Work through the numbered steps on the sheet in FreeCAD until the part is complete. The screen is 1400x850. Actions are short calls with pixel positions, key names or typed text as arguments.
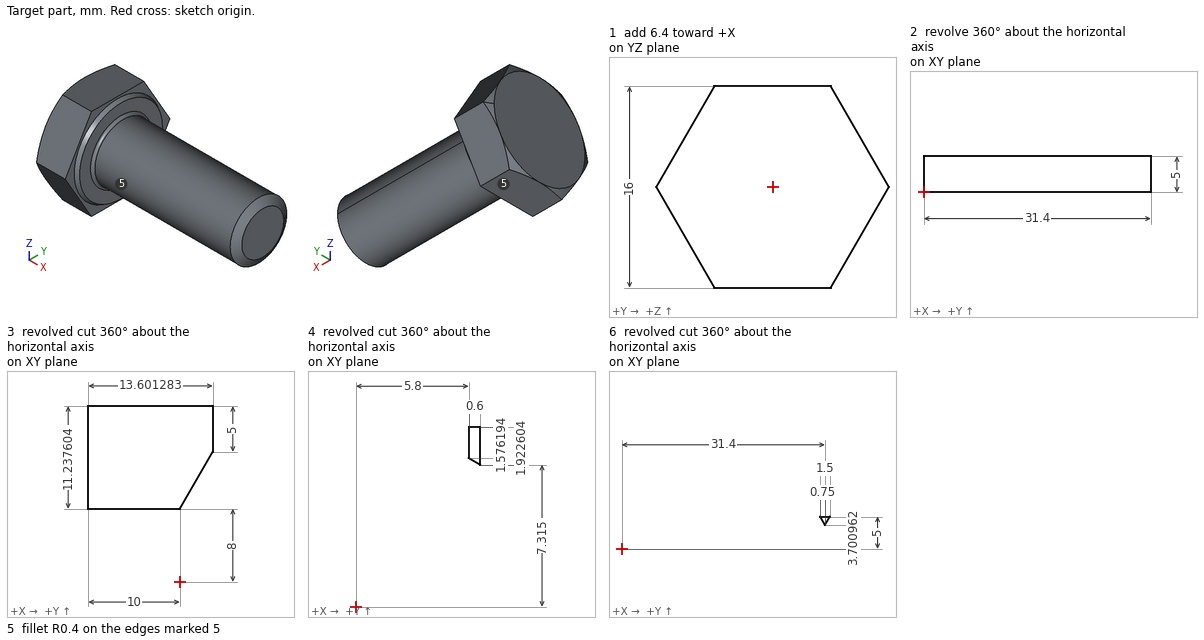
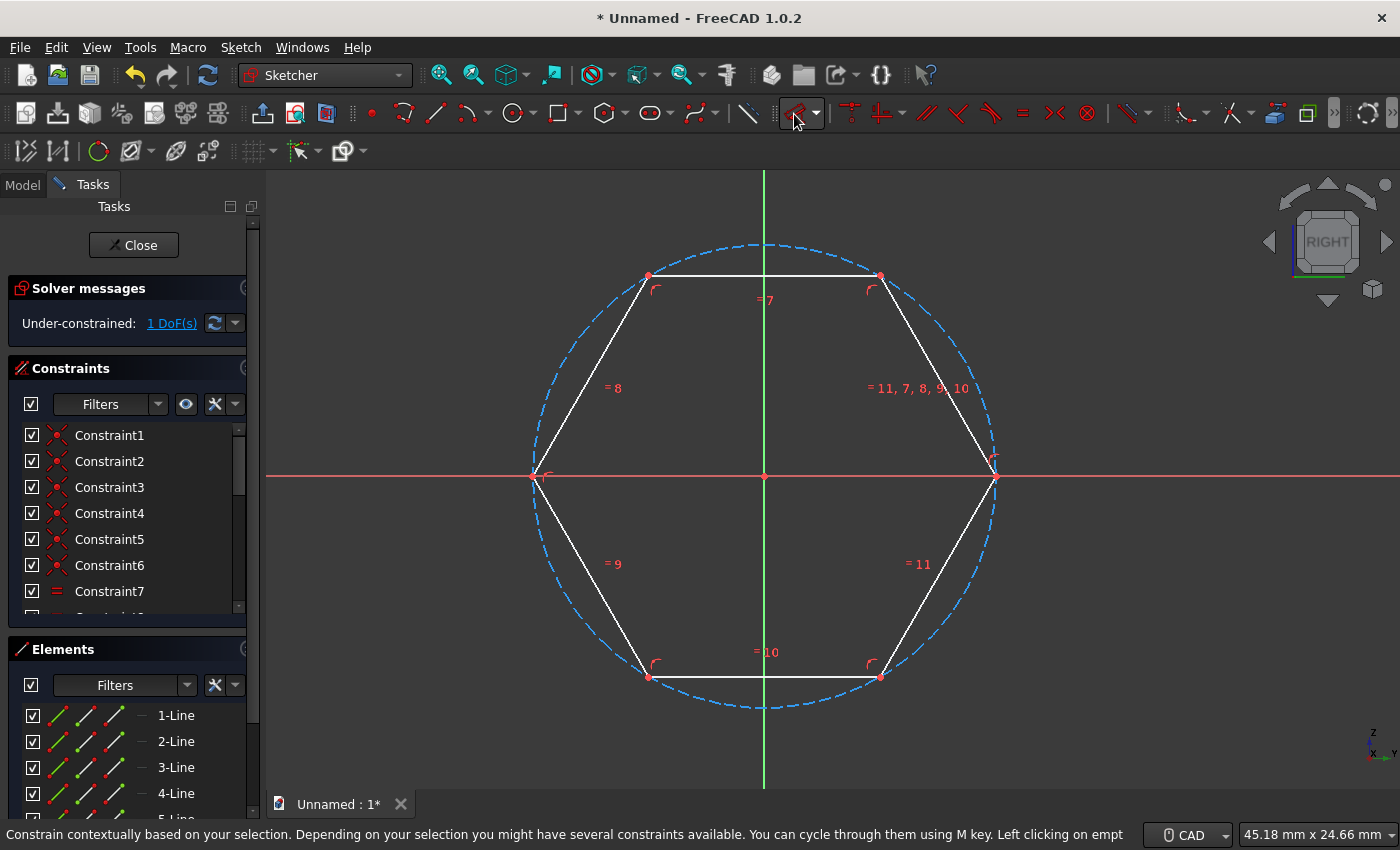
click(649, 677)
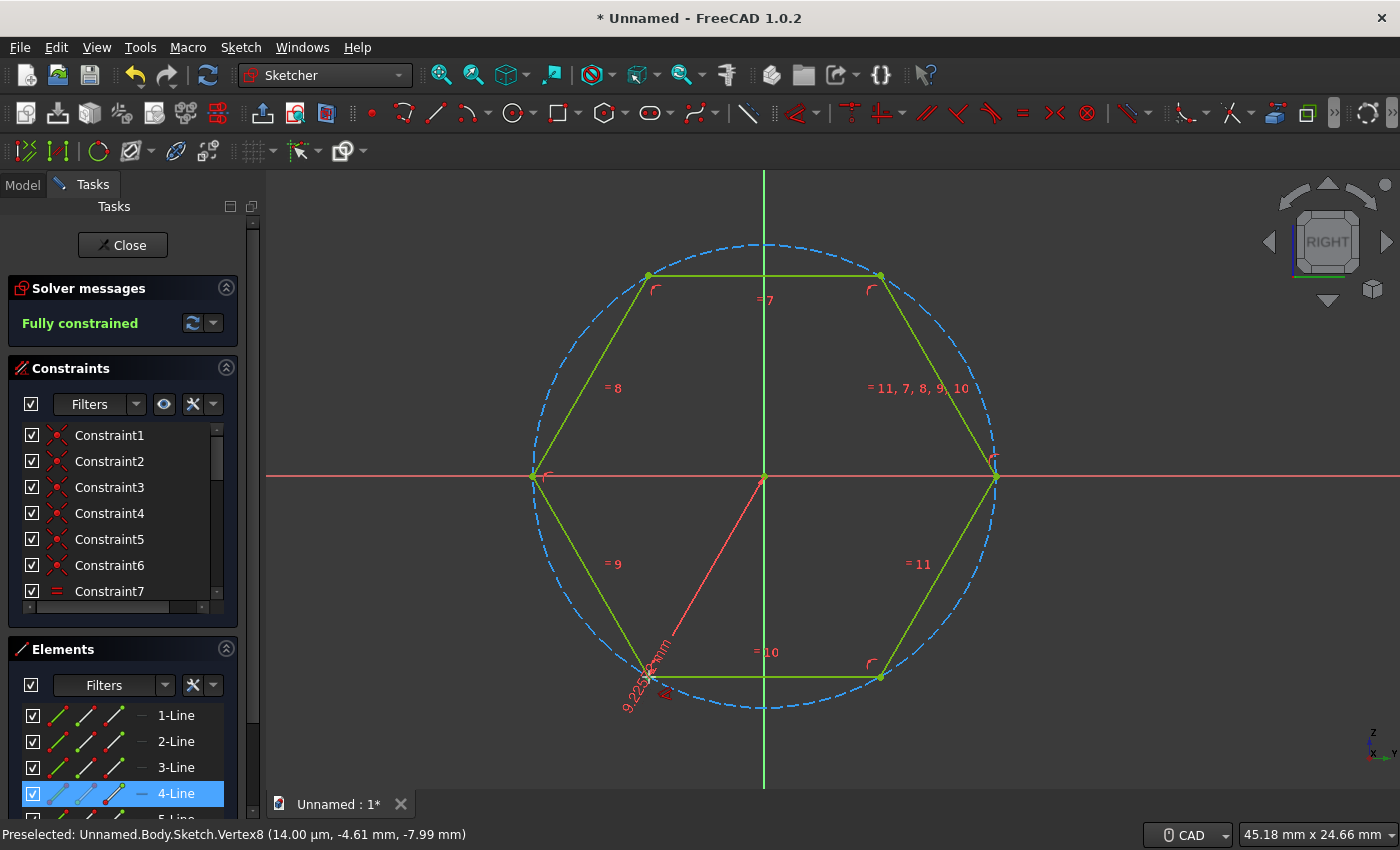
click(880, 276)
click(914, 384)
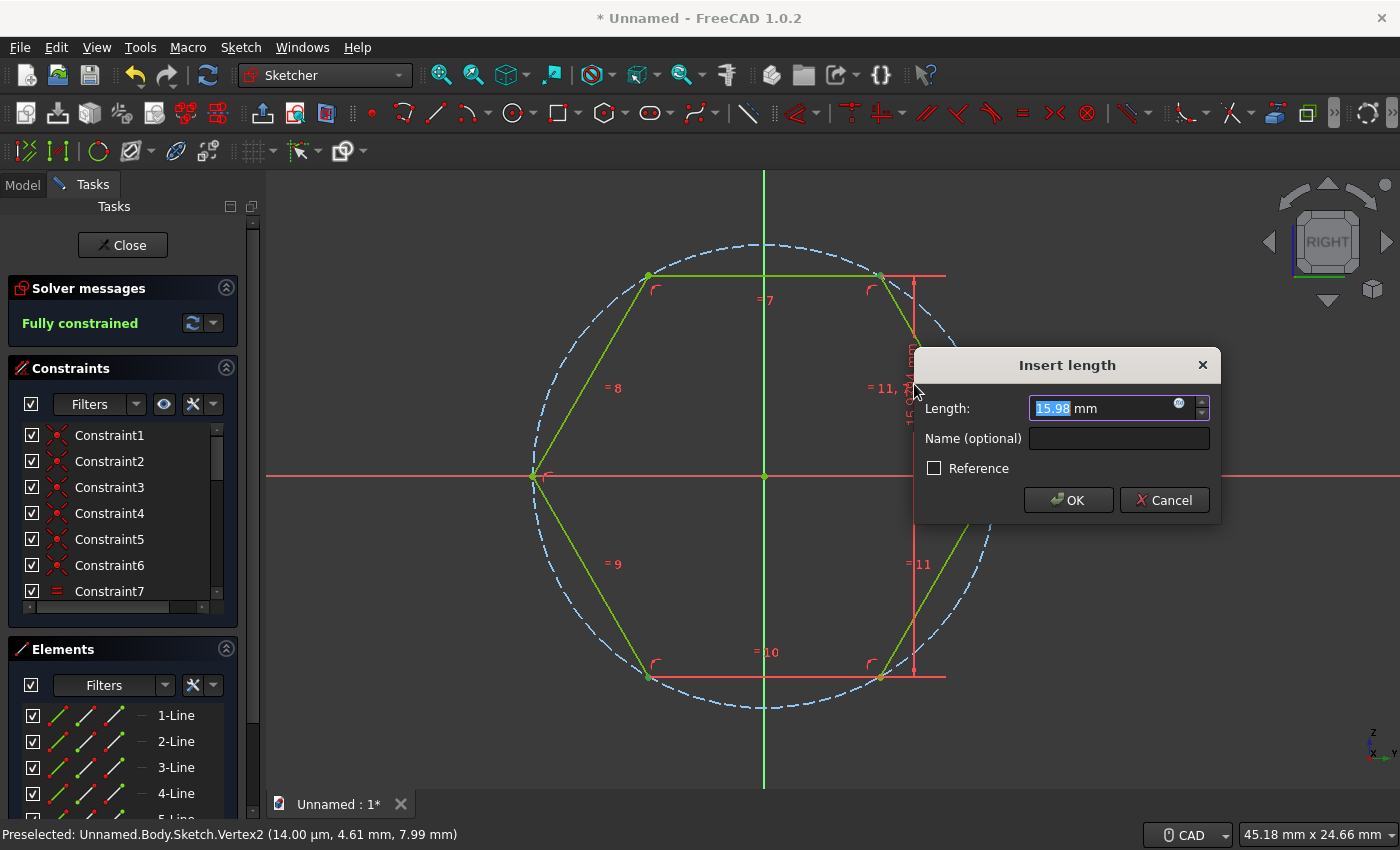
text(16)
key(Return)
key(Escape)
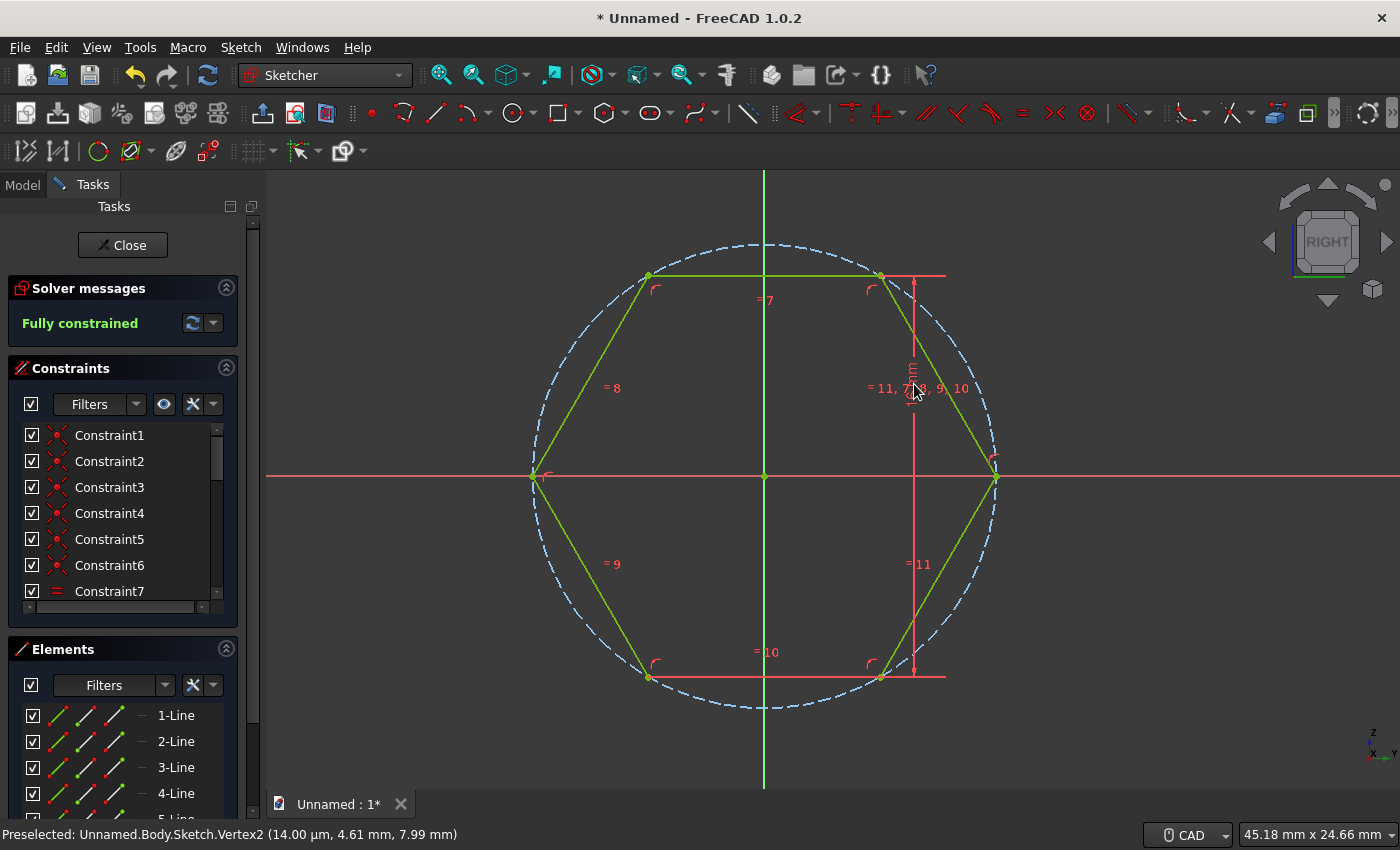
click(123, 245)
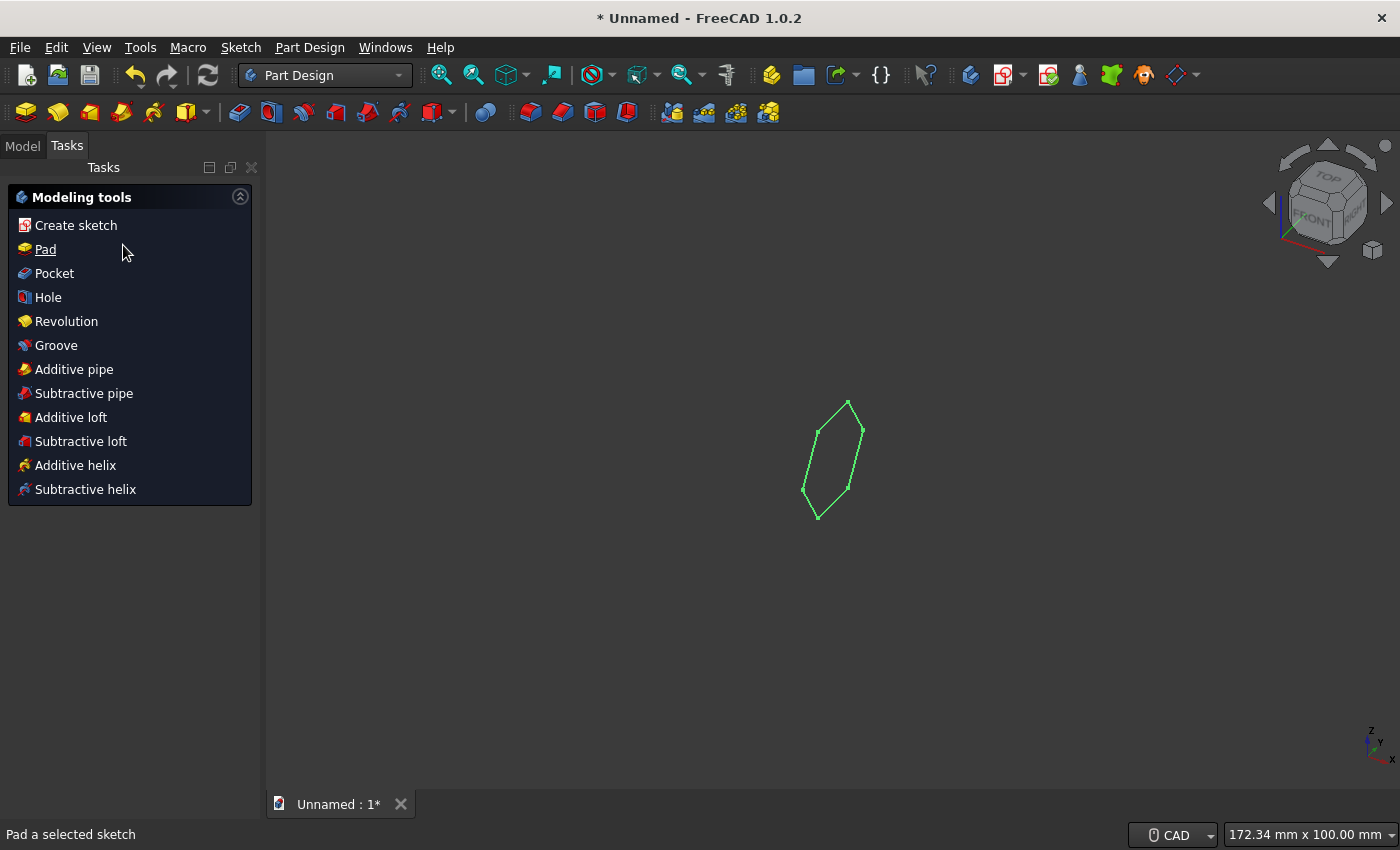
click(26, 112)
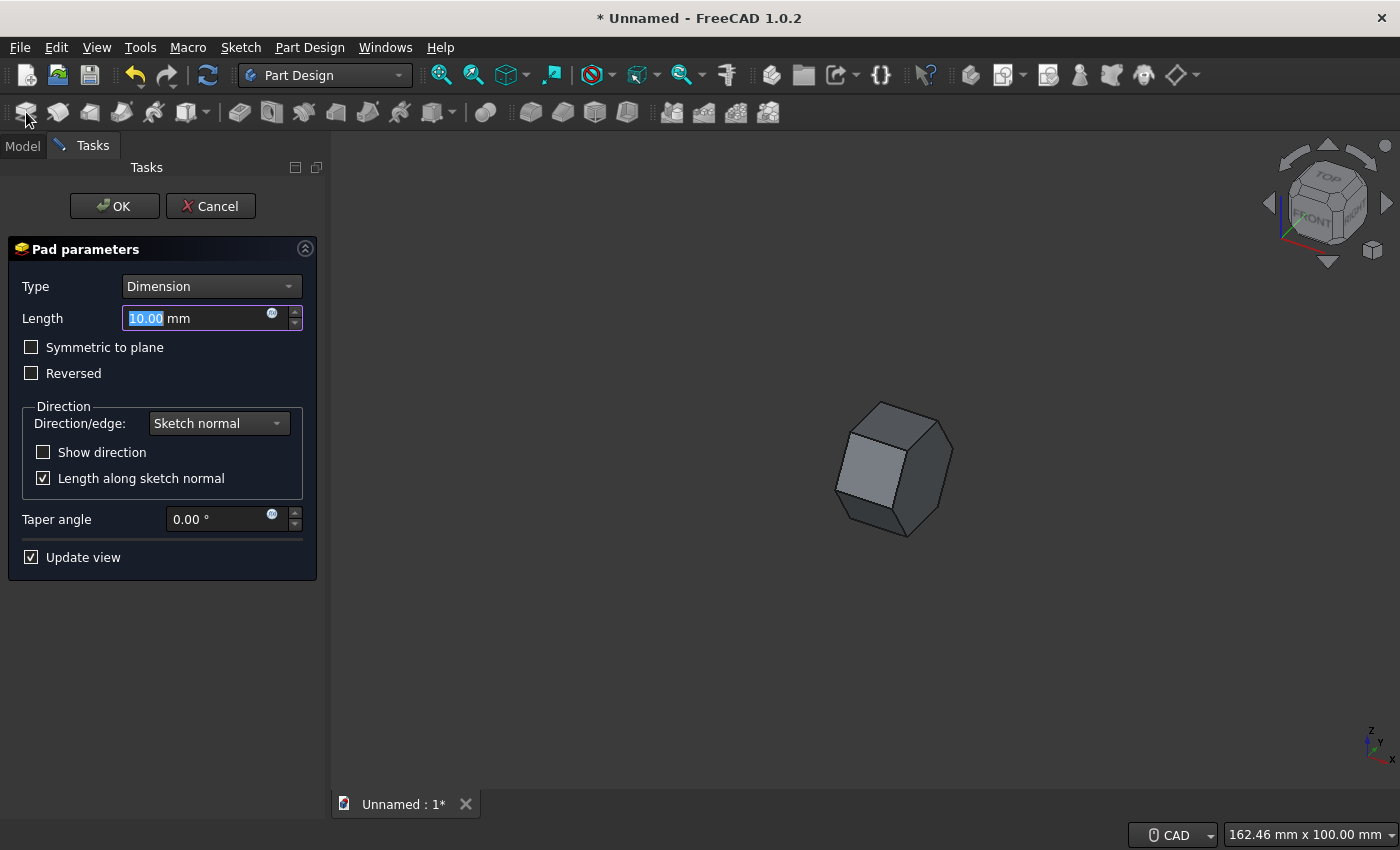
text(6.4)
key(Tab)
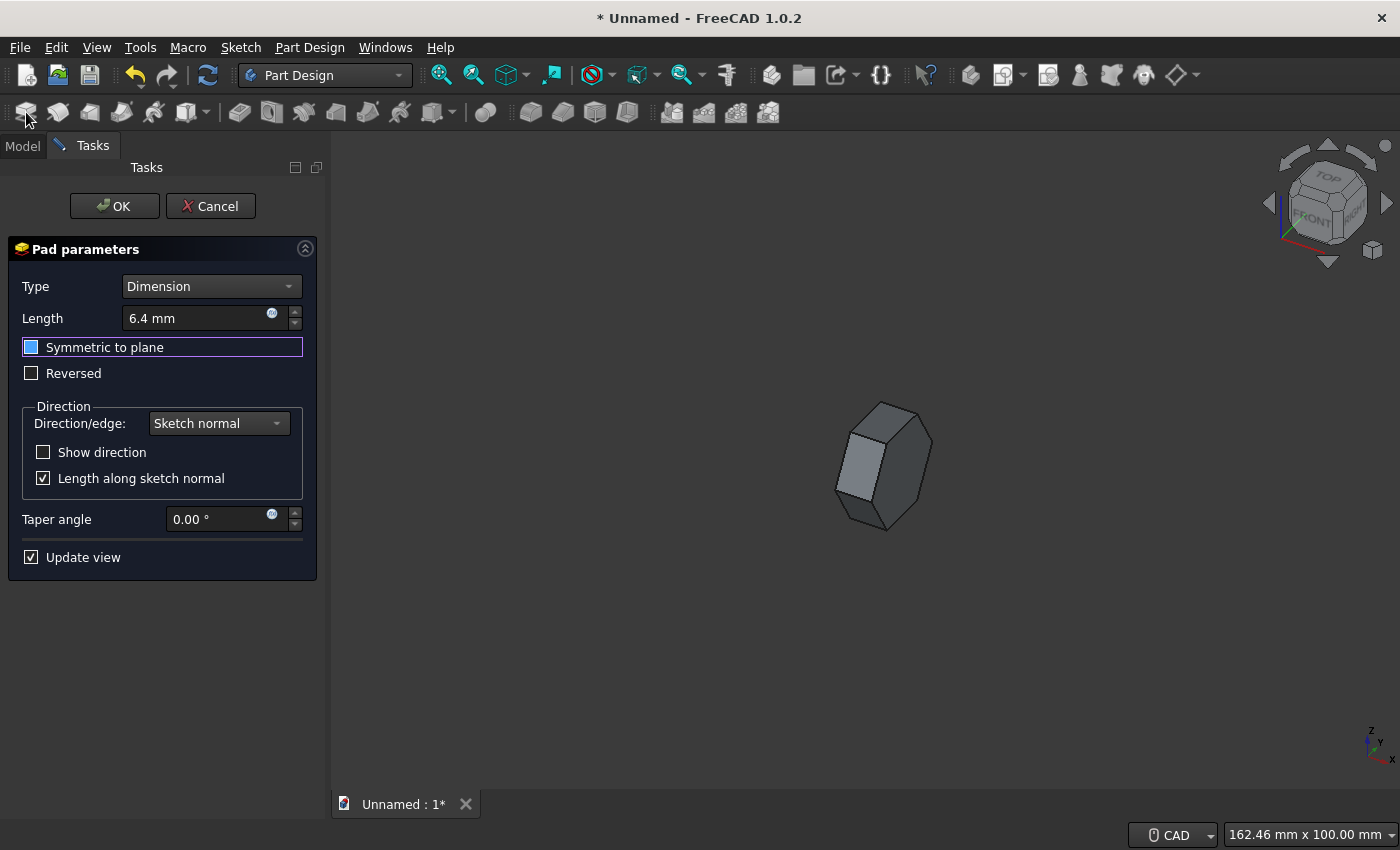
click(115, 206)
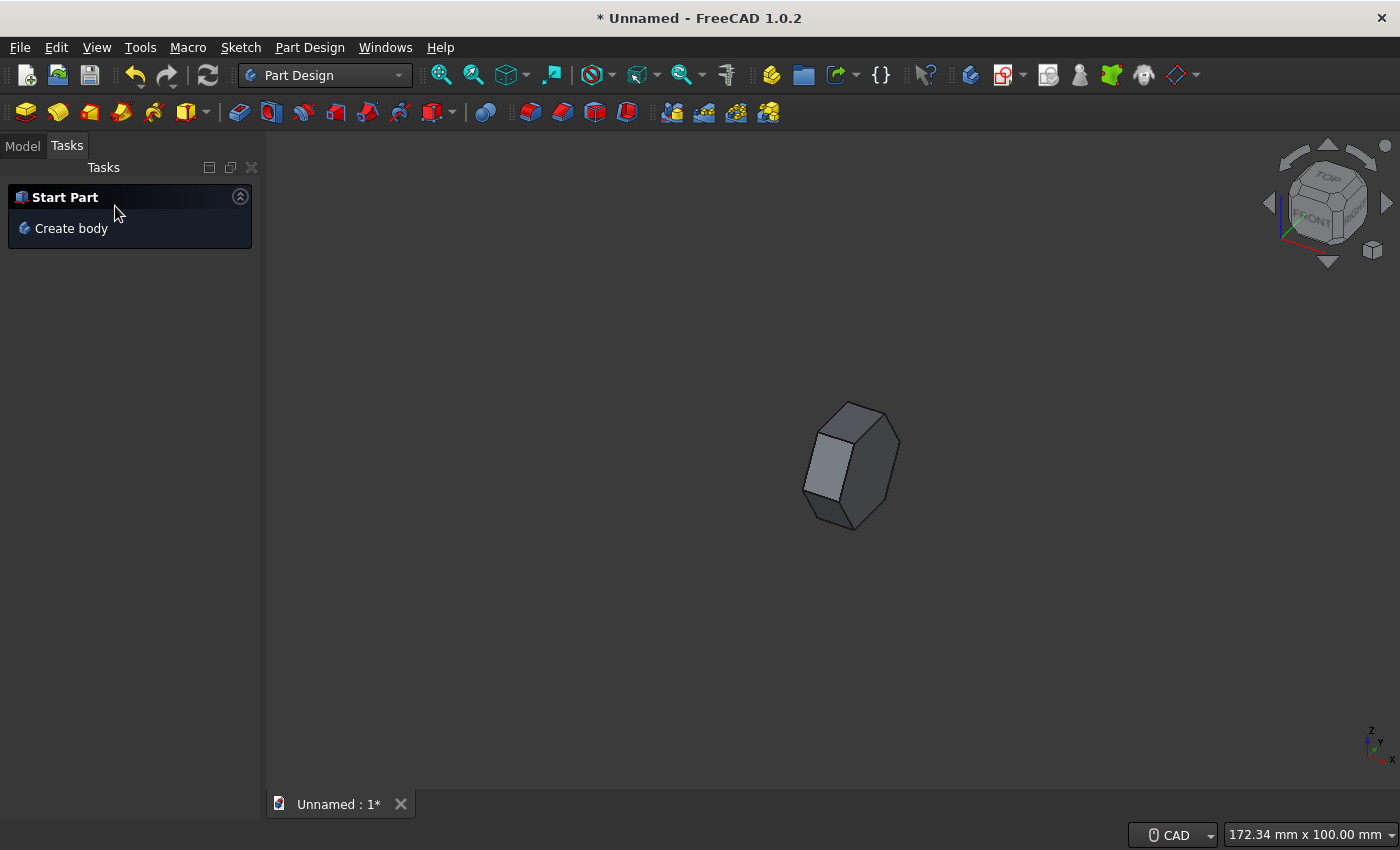
click(442, 76)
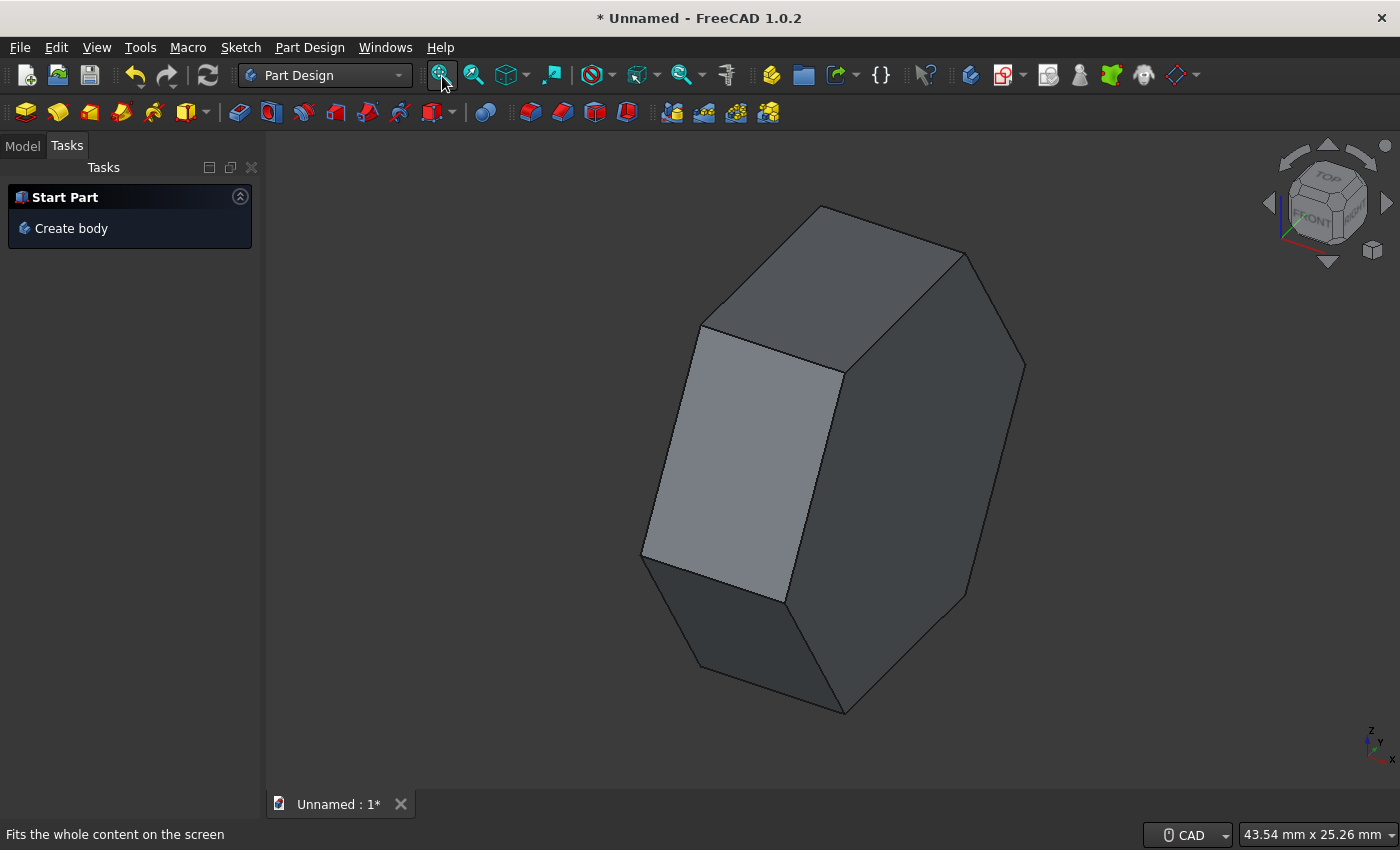
click(1004, 76)